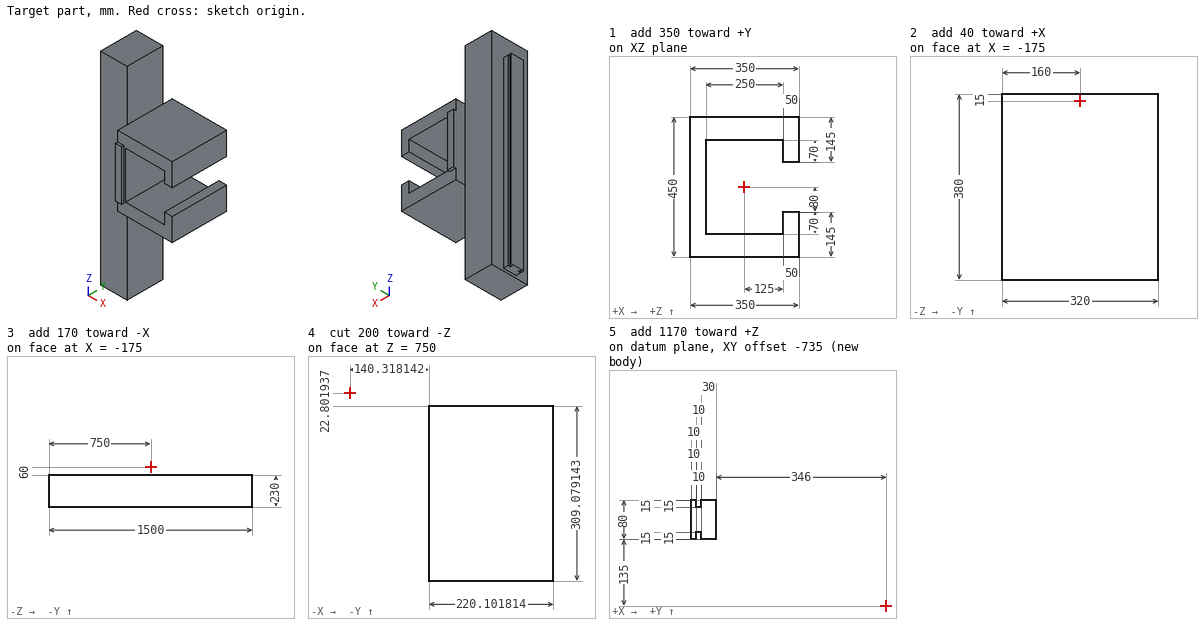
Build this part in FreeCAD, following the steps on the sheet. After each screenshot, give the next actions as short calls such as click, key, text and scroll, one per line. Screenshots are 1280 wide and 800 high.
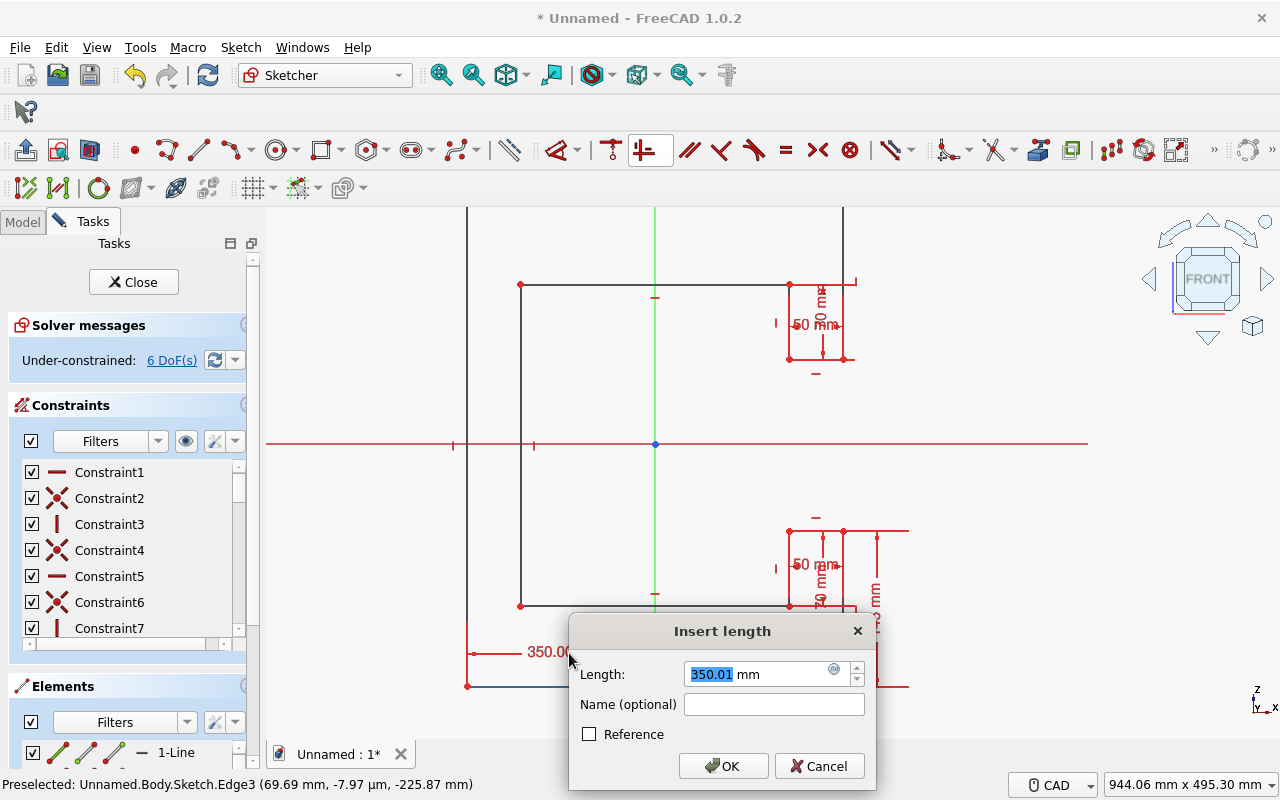
text(350)
key(Return)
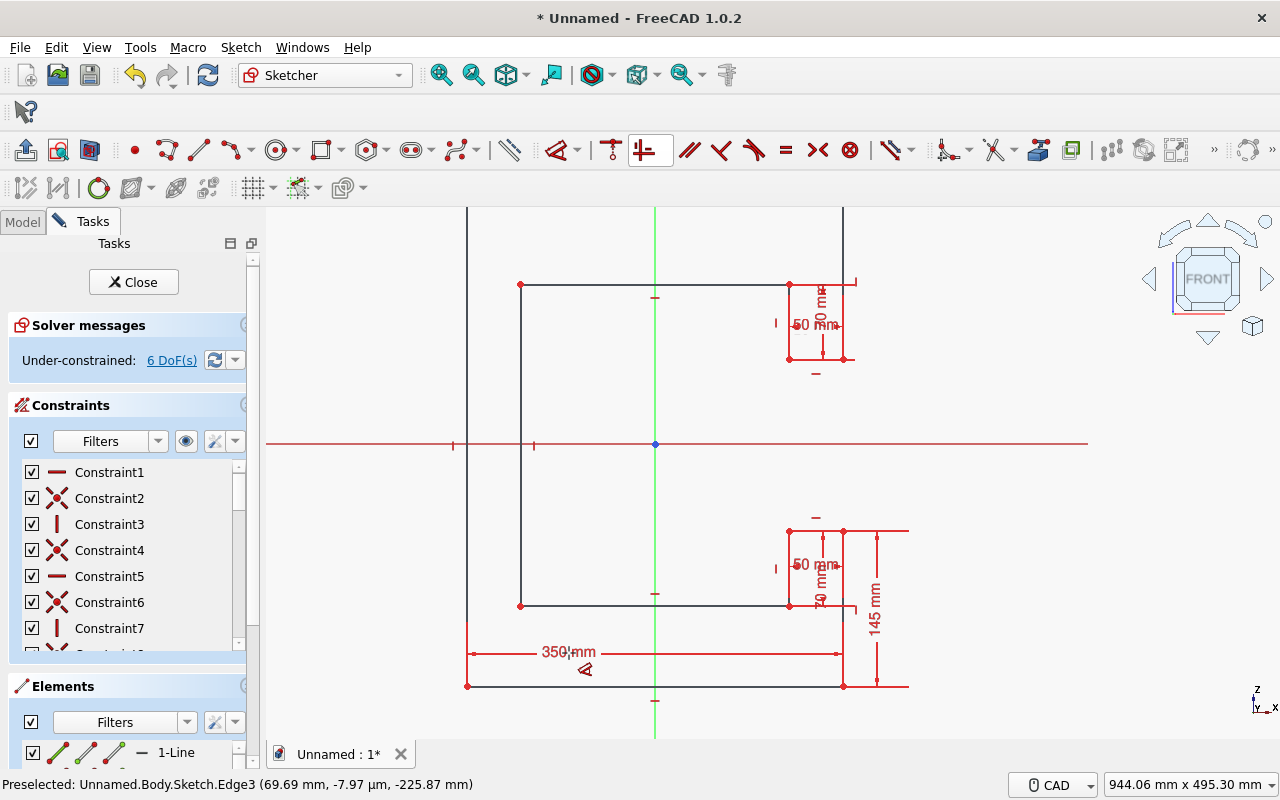
click(467, 542)
click(433, 461)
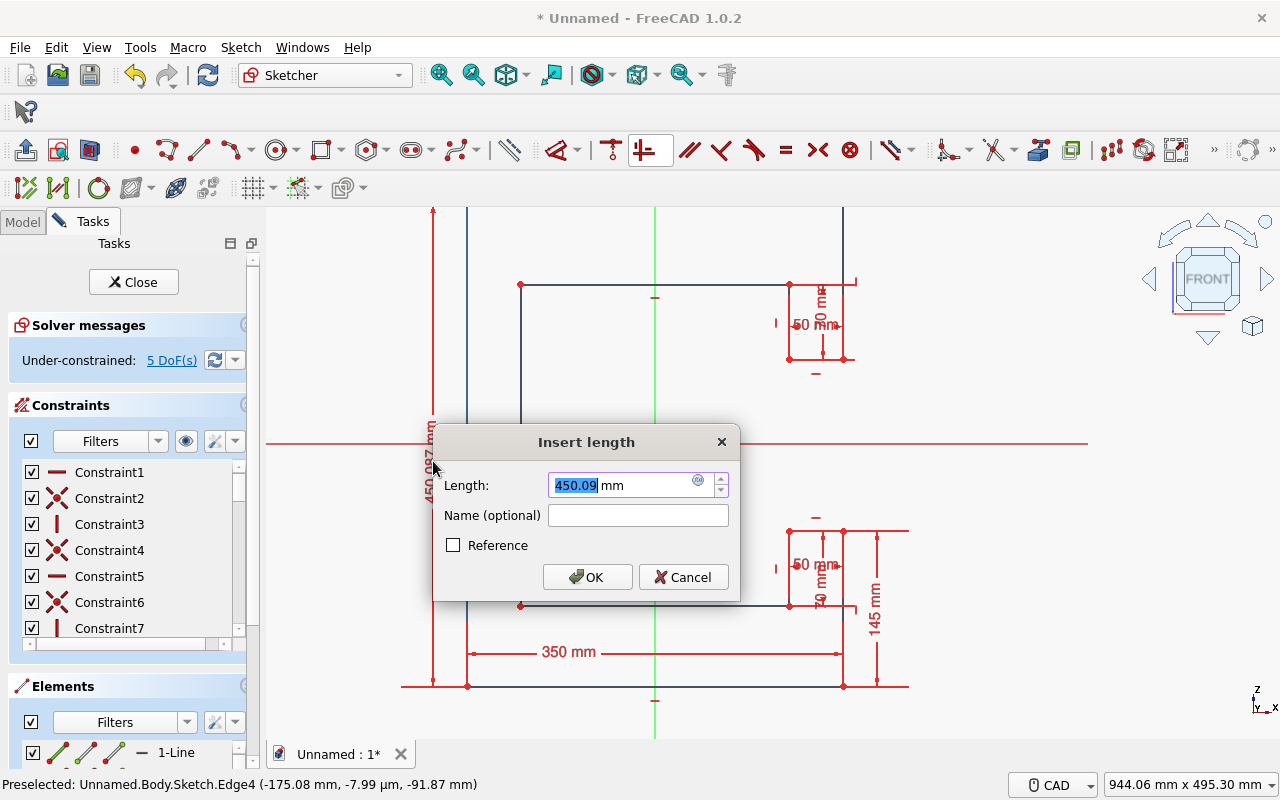
text(450)
key(Return)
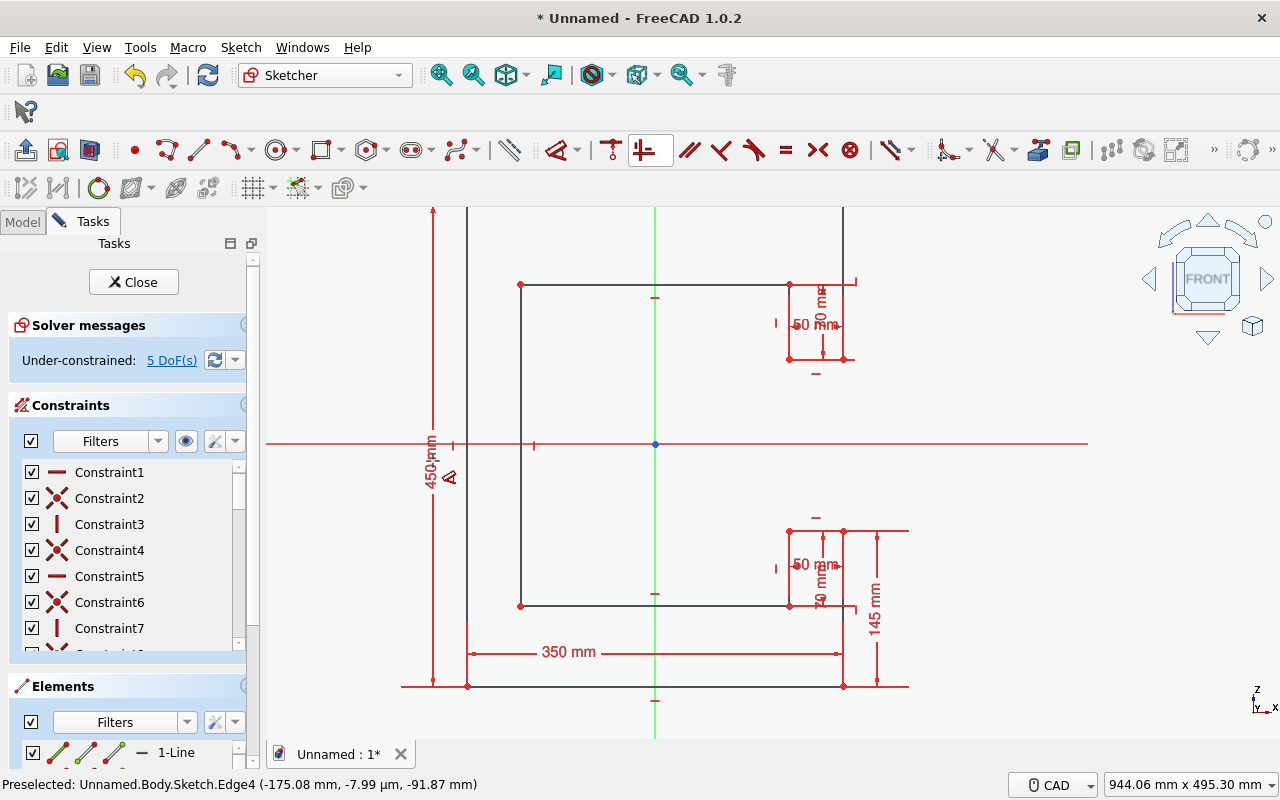
scroll(805, 531, down, 2)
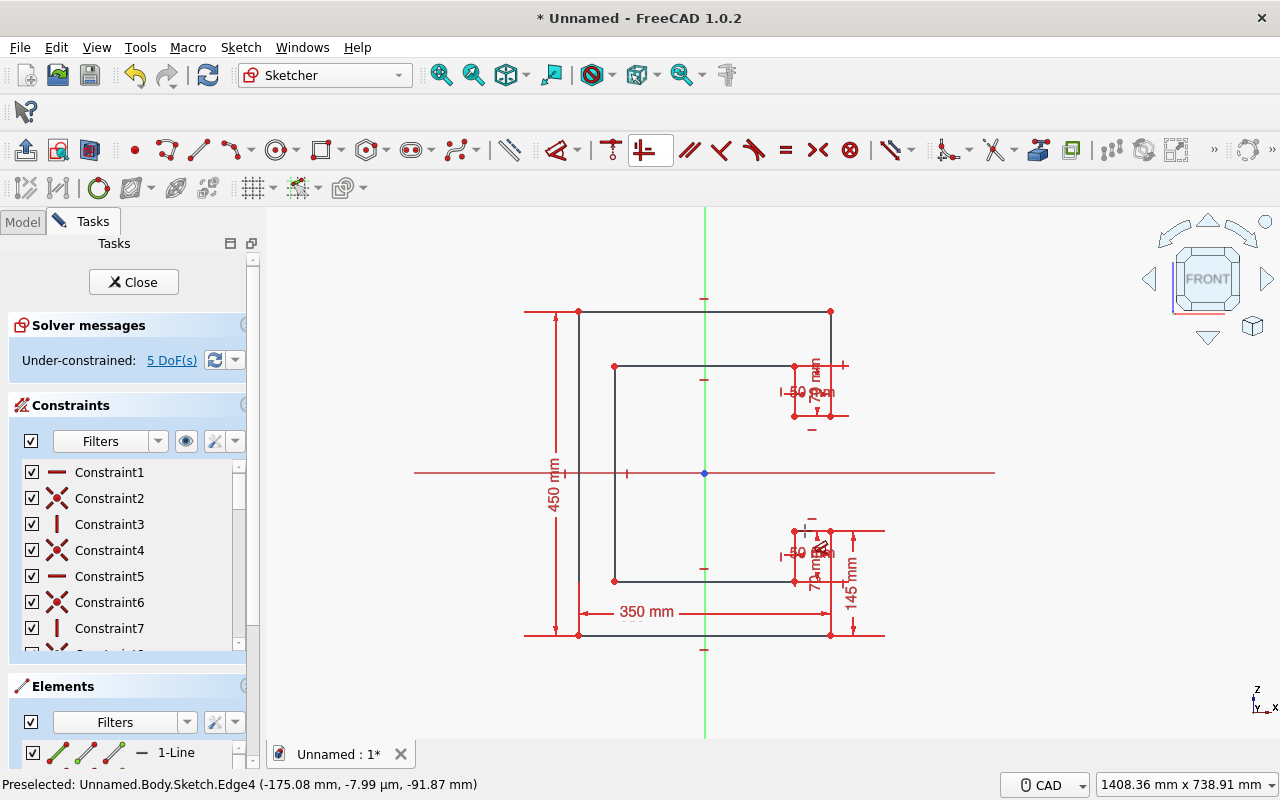
click(654, 312)
click(647, 278)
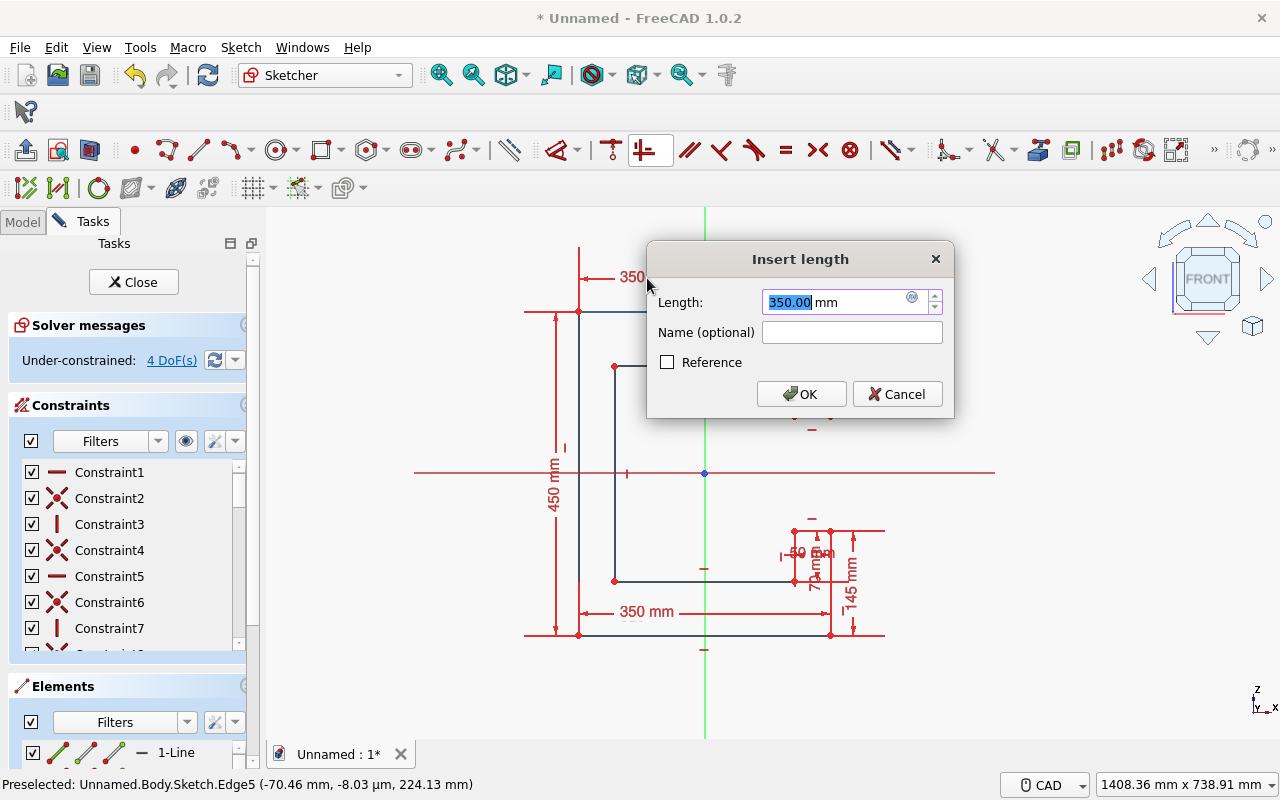
text(350)
key(Return)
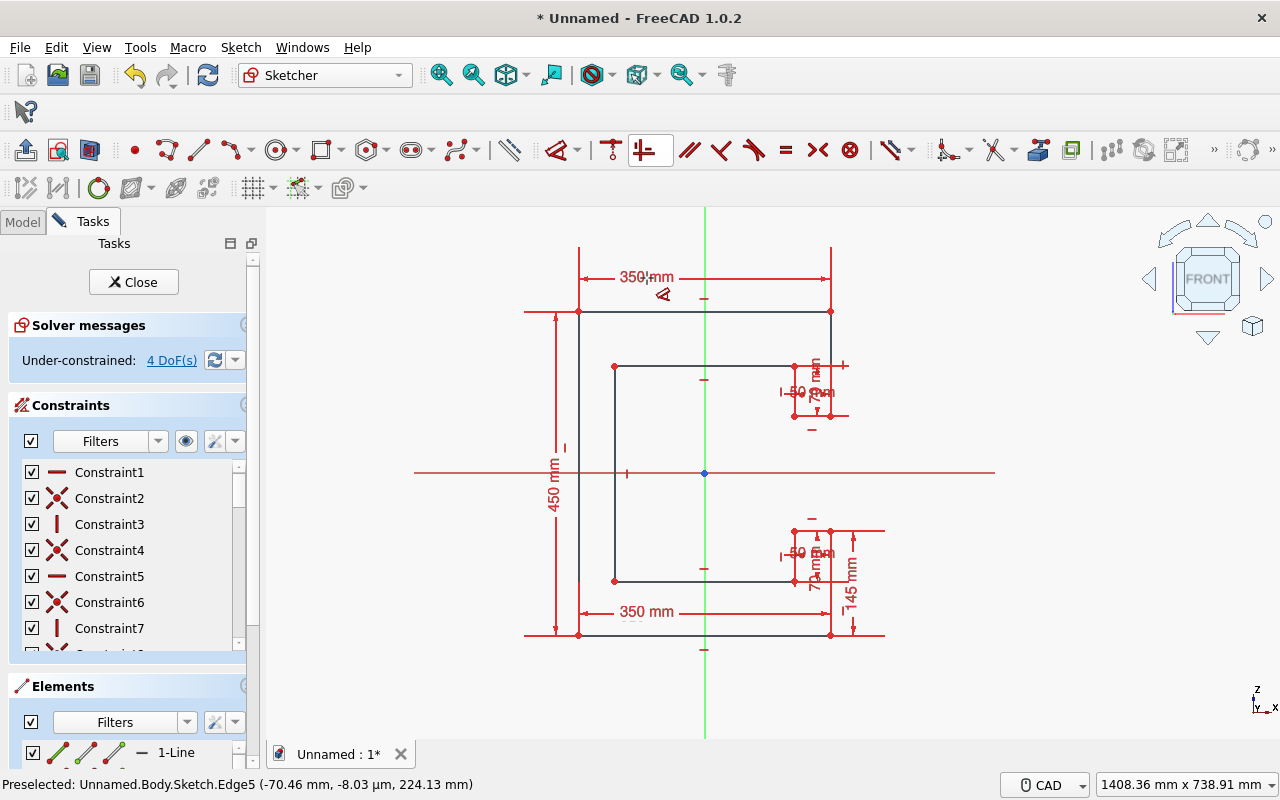
click(831, 343)
click(865, 340)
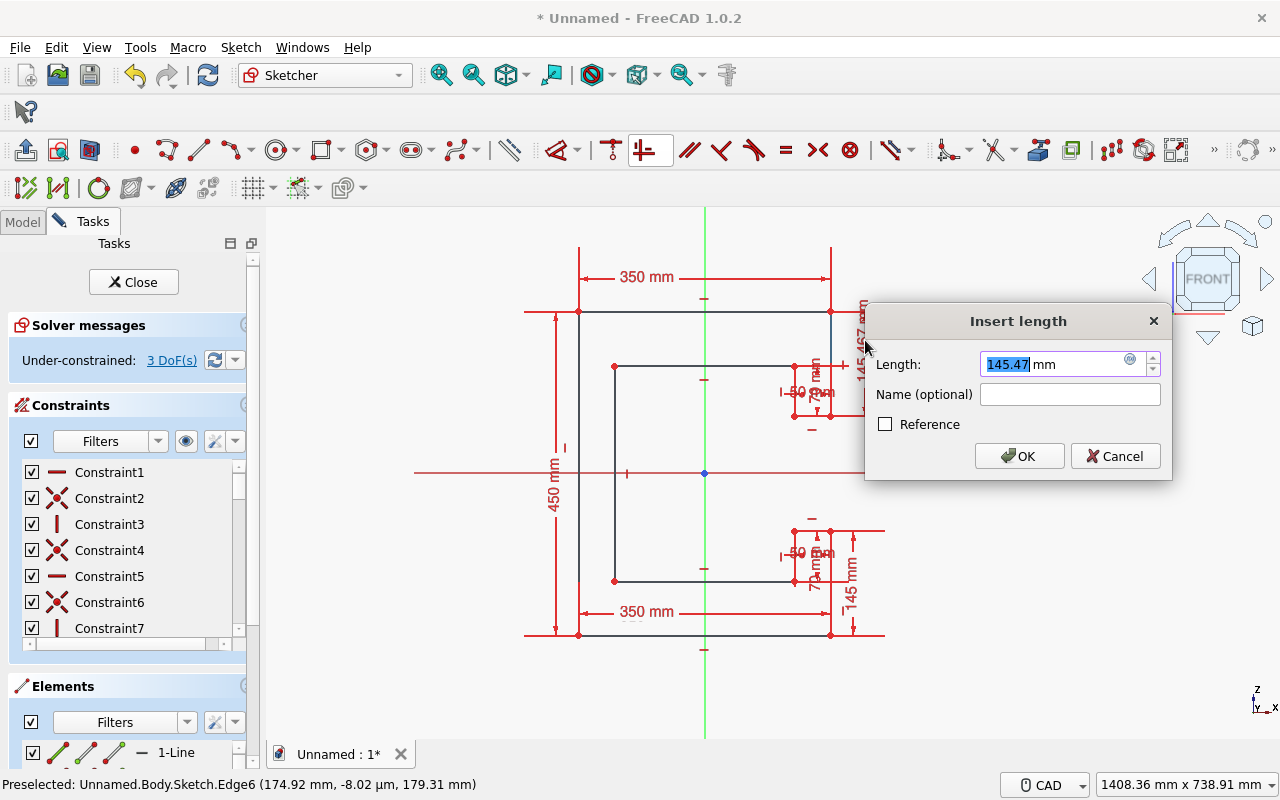
text(145)
key(Return)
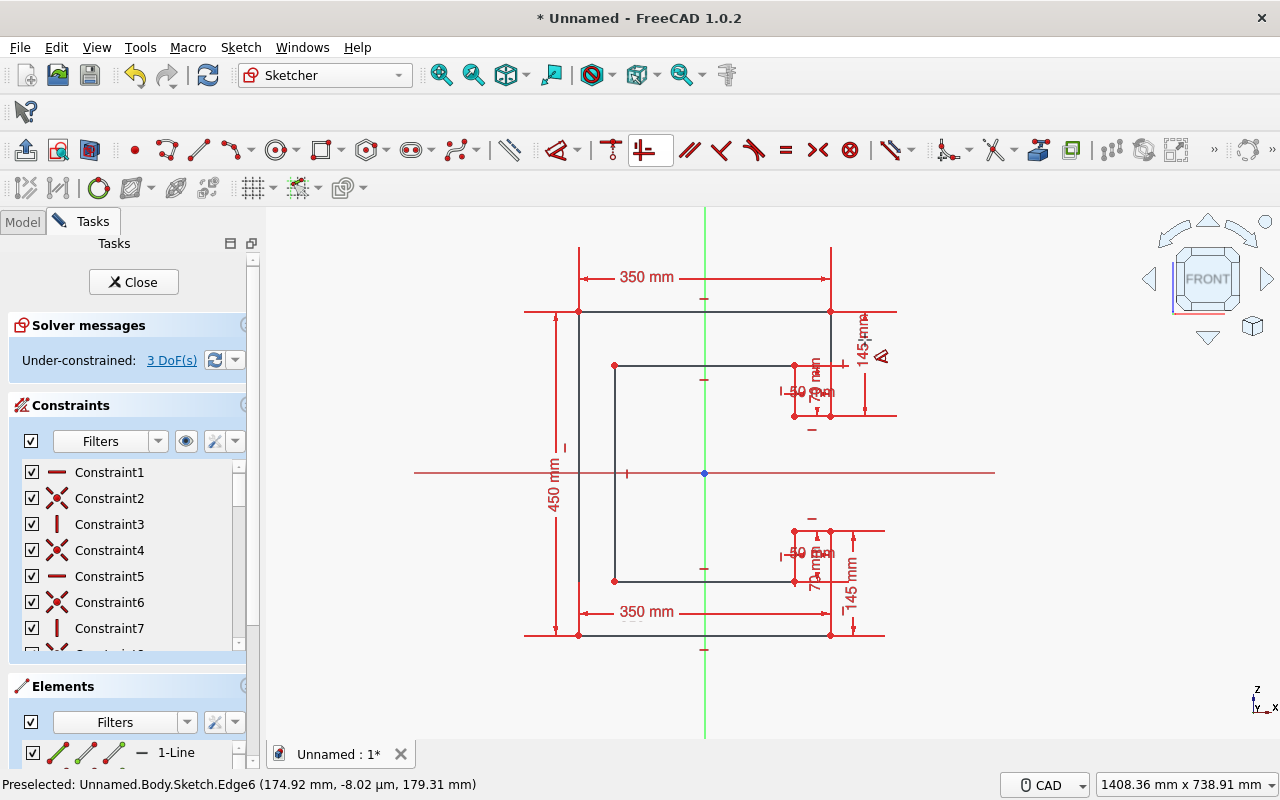
click(741, 366)
click(663, 332)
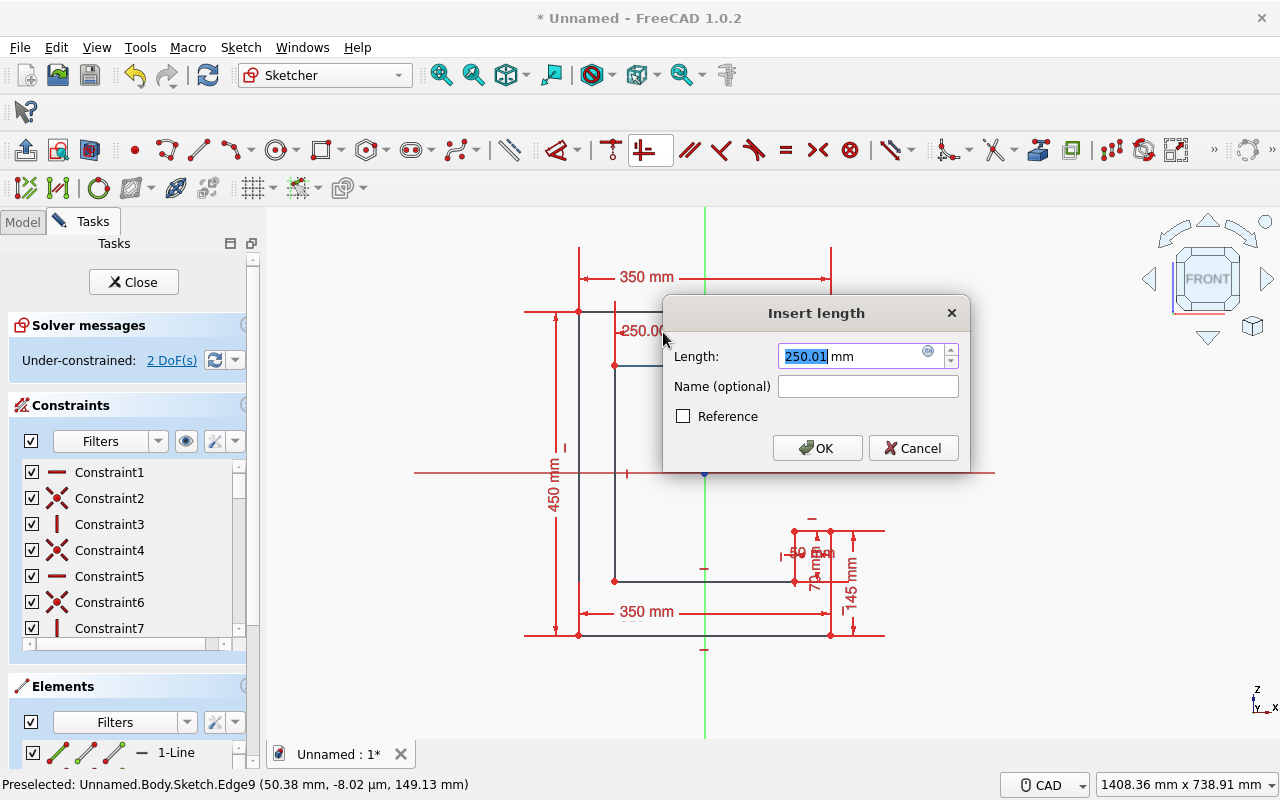
text(250)
key(Return)